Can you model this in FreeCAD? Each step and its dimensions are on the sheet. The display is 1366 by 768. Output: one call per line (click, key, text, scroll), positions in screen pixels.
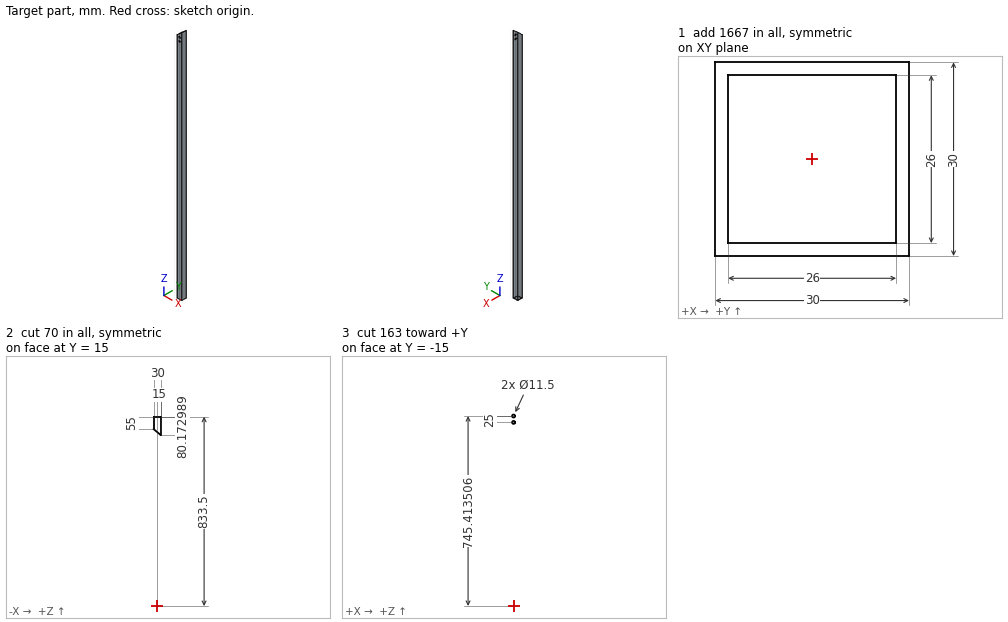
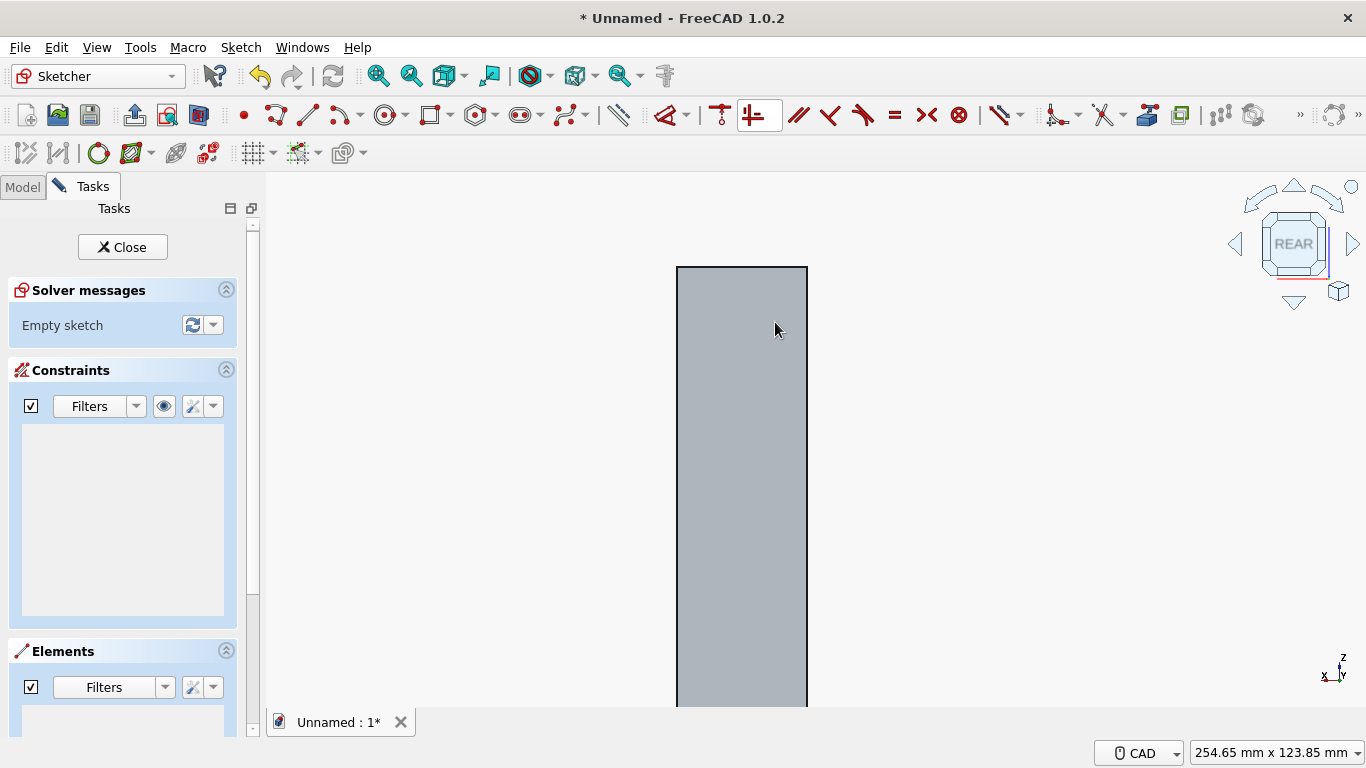
click(276, 116)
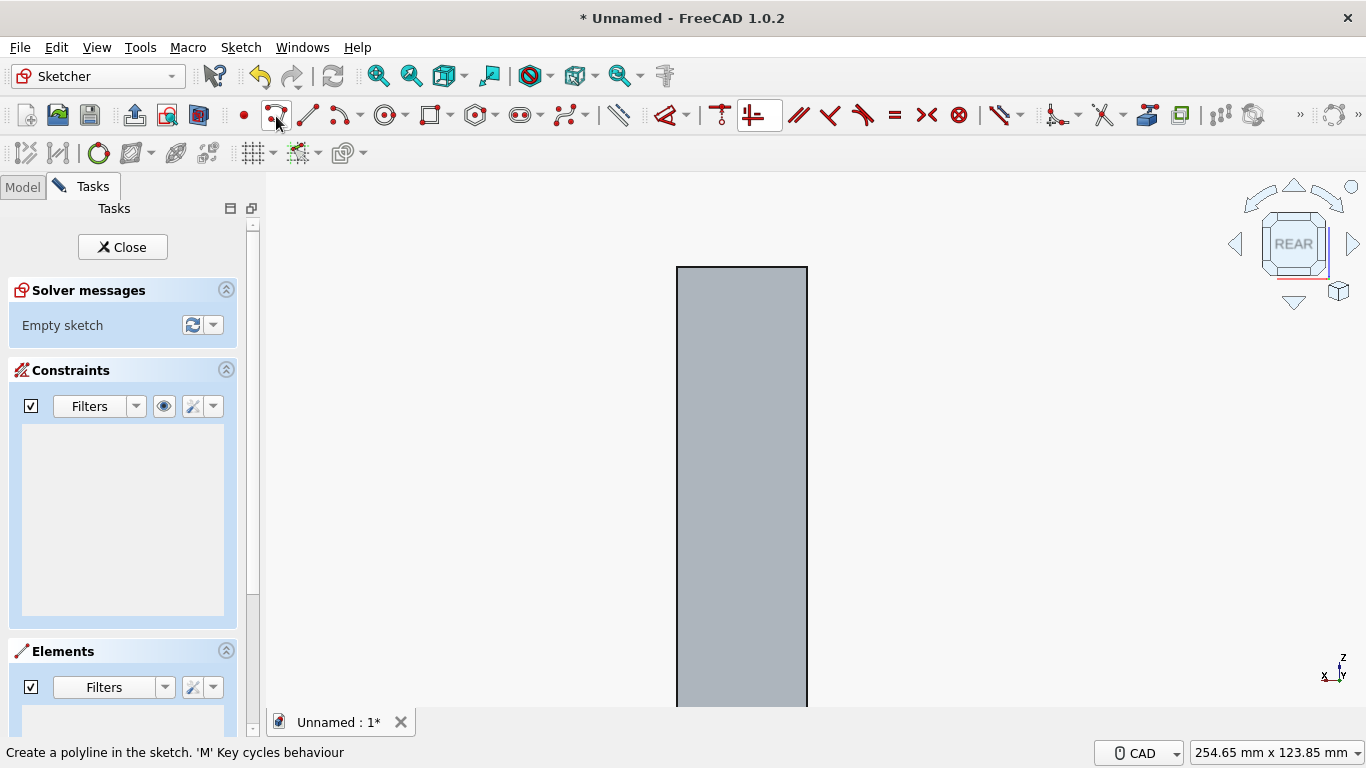
click(807, 614)
click(807, 267)
click(677, 267)
click(677, 505)
click(807, 615)
key(Escape)
key(Escape)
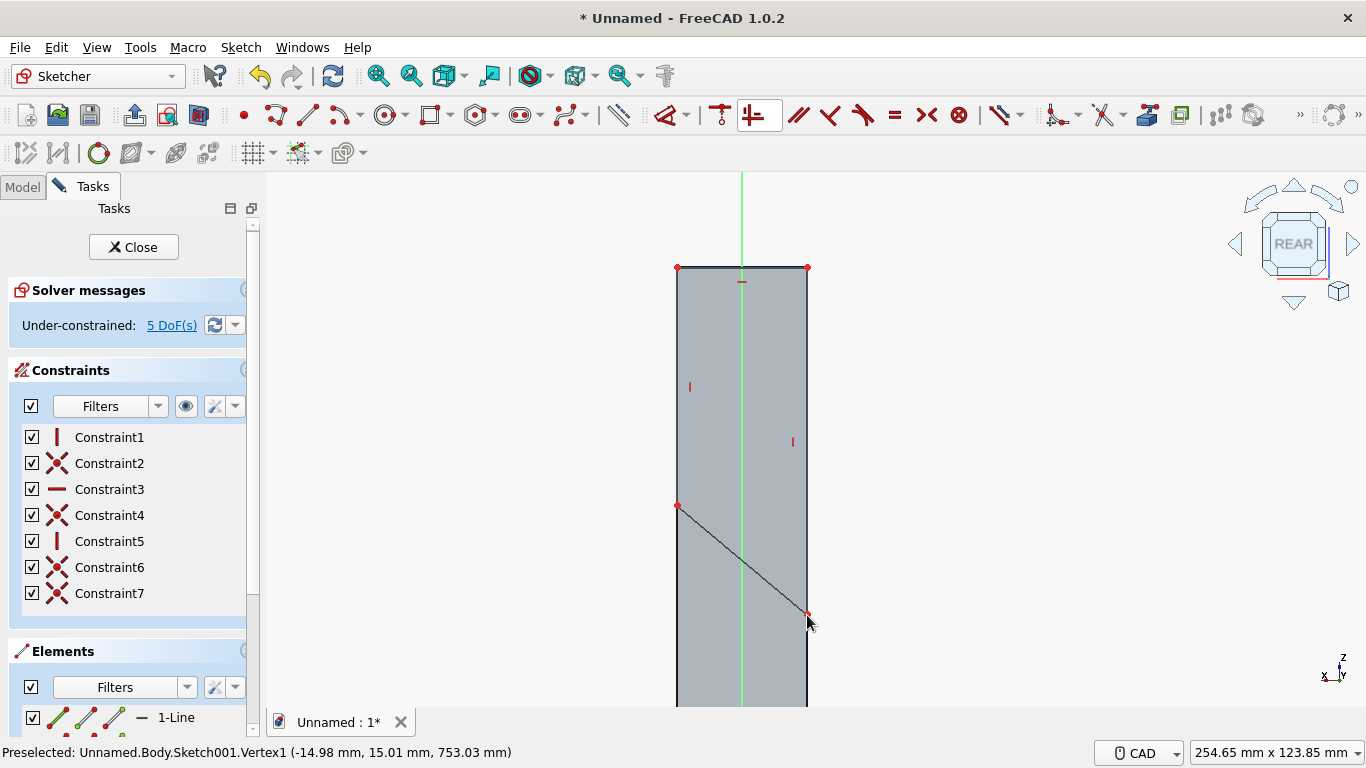
click(666, 116)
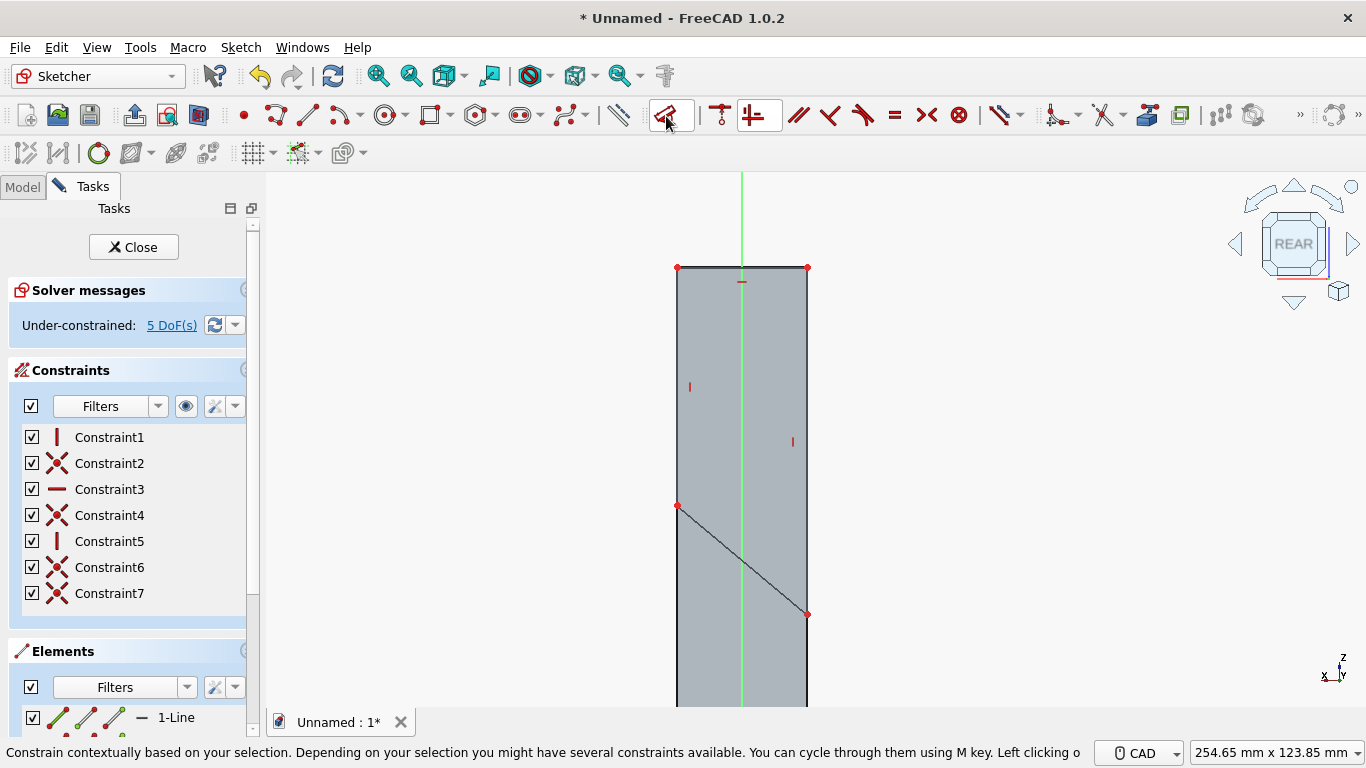
click(768, 268)
click(712, 234)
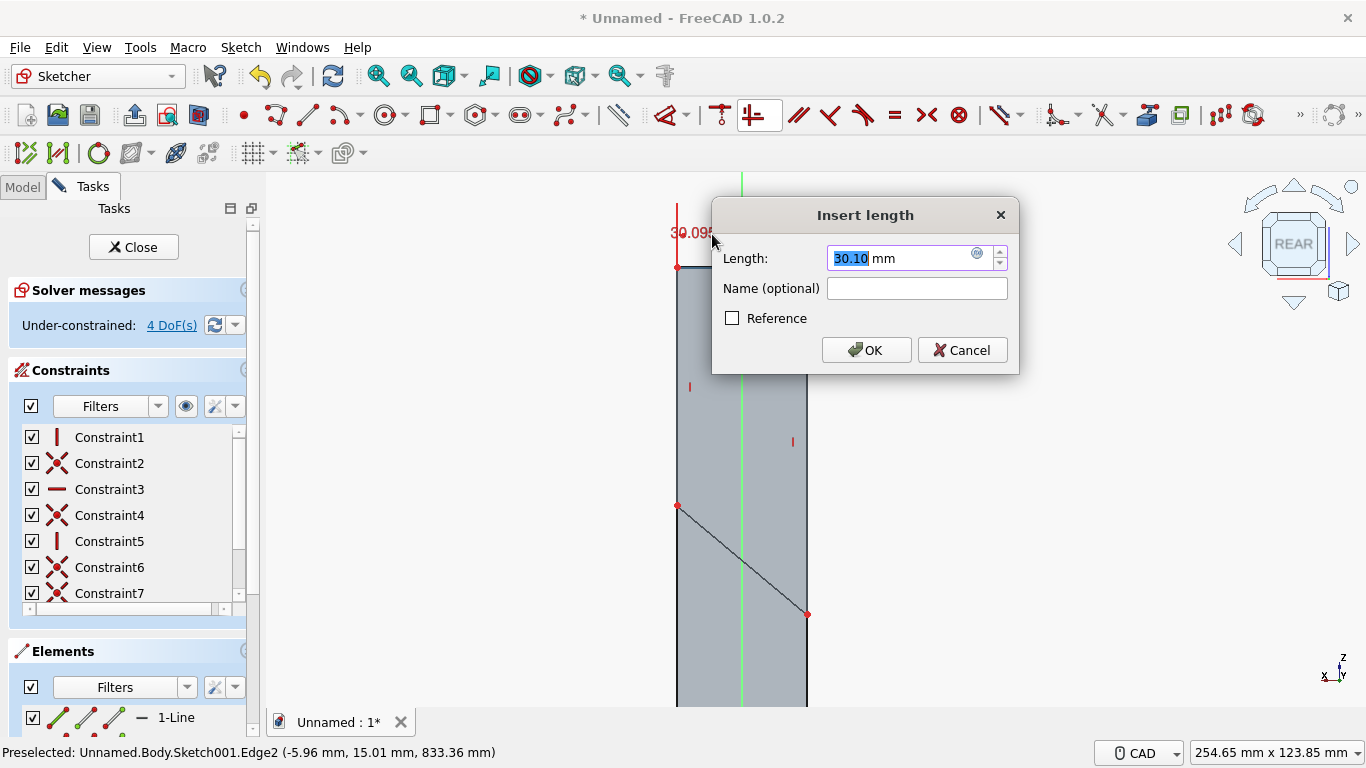
text(30)
key(Return)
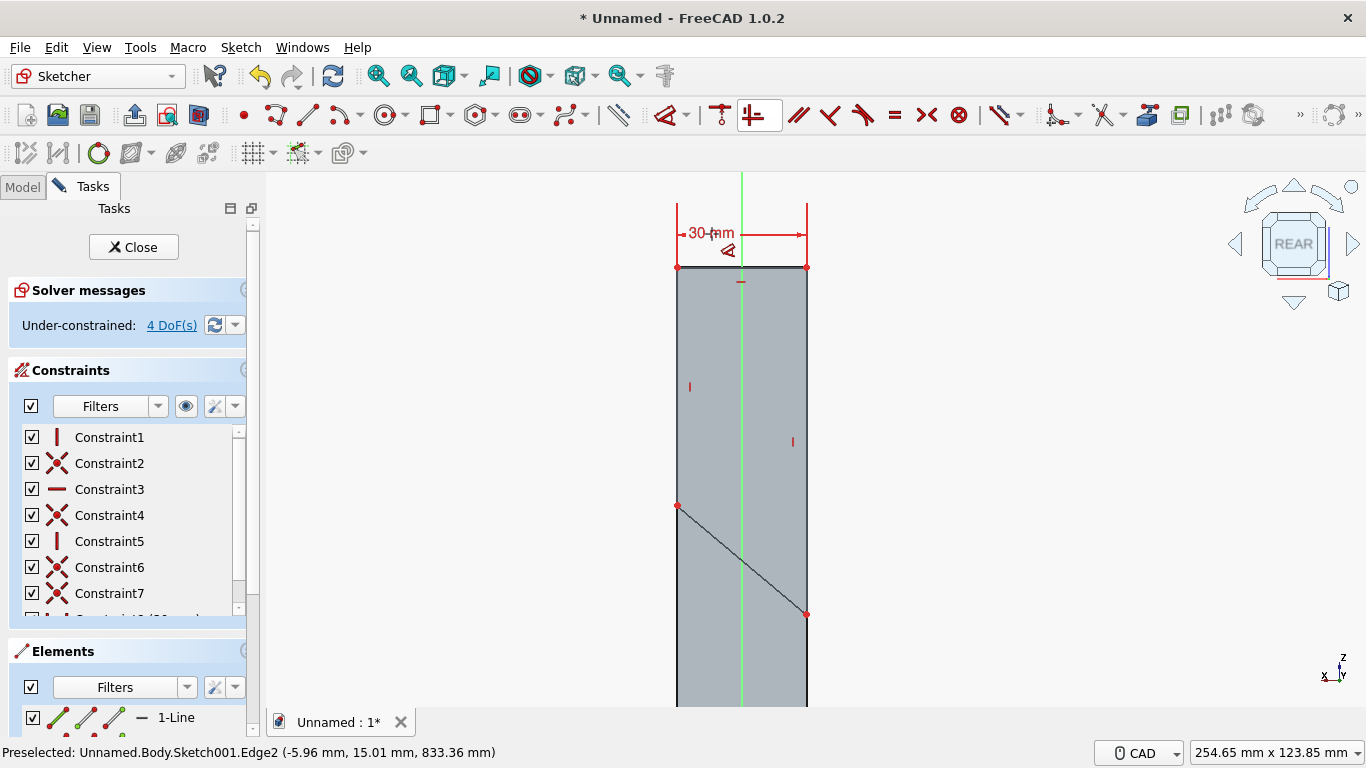
click(677, 339)
click(643, 387)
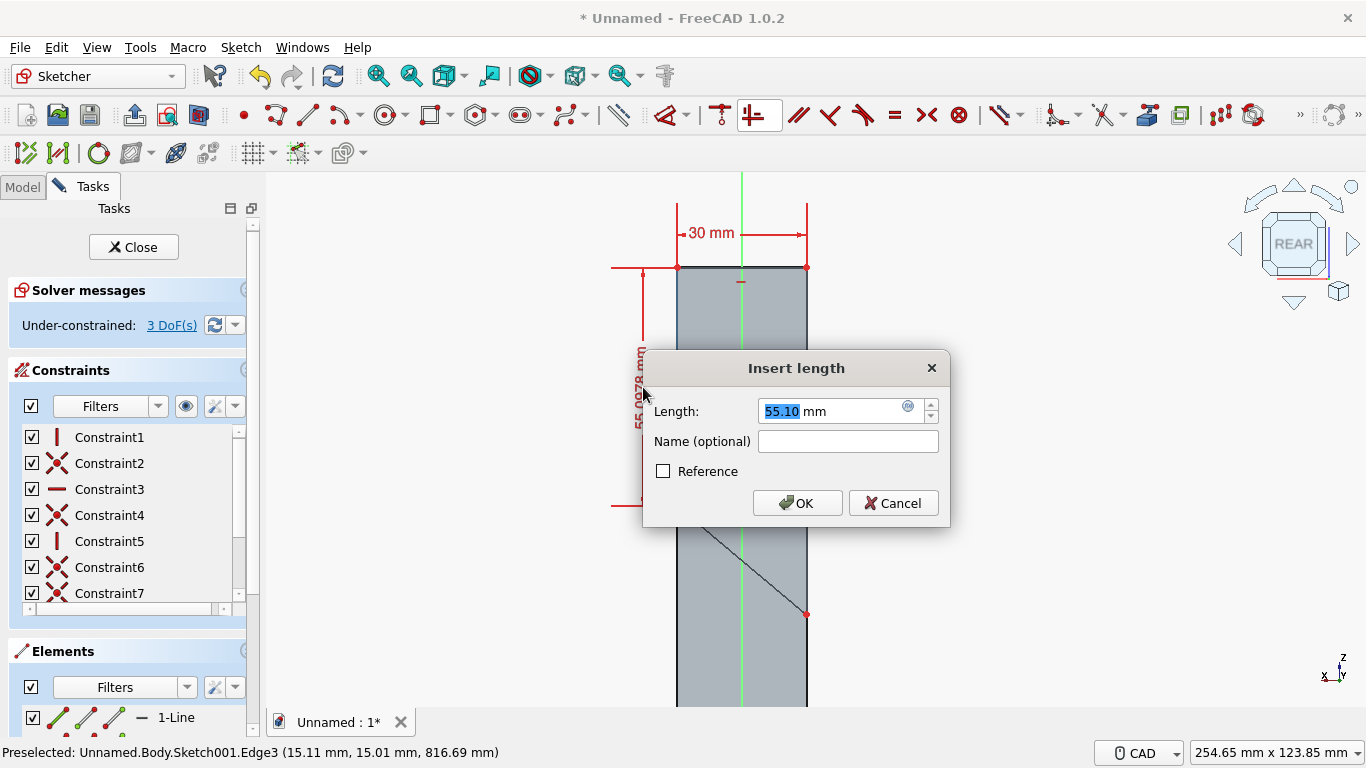
text(55)
key(Return)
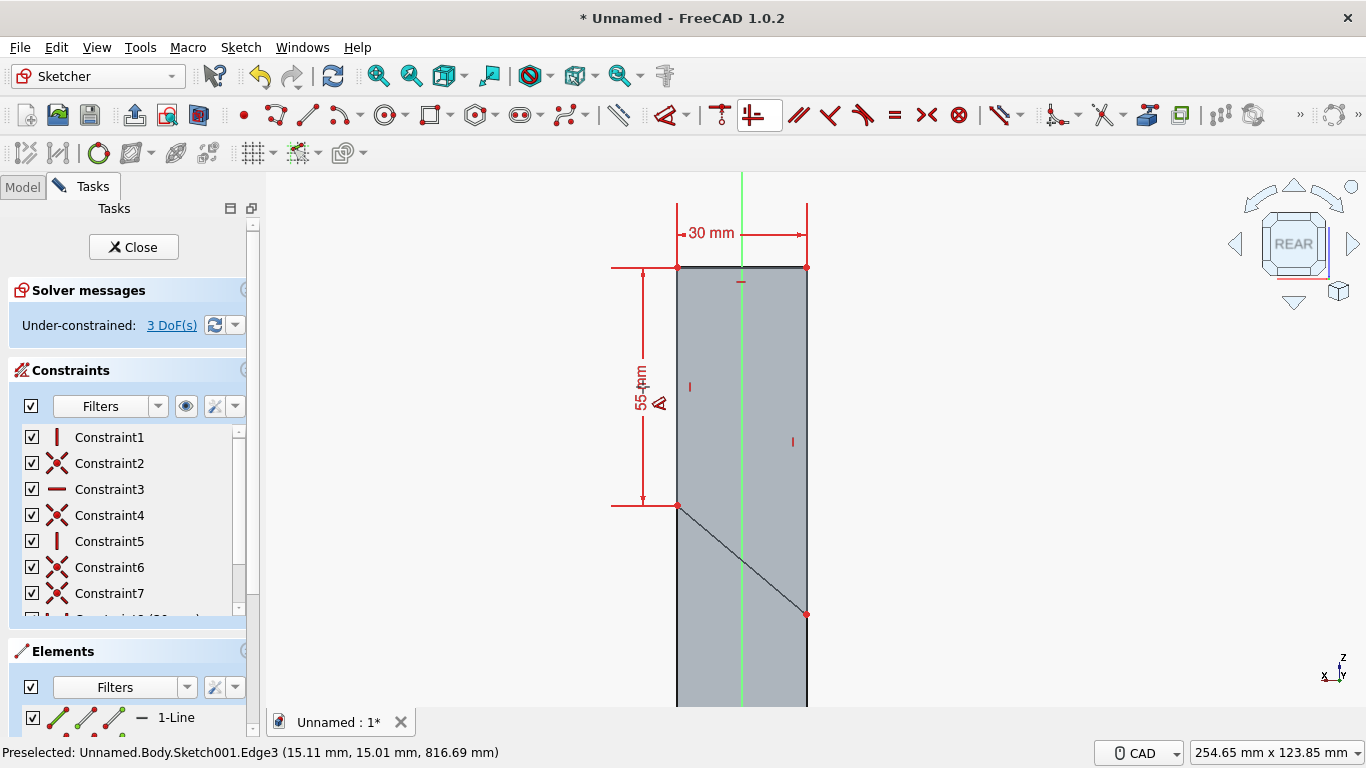
click(807, 615)
click(789, 581)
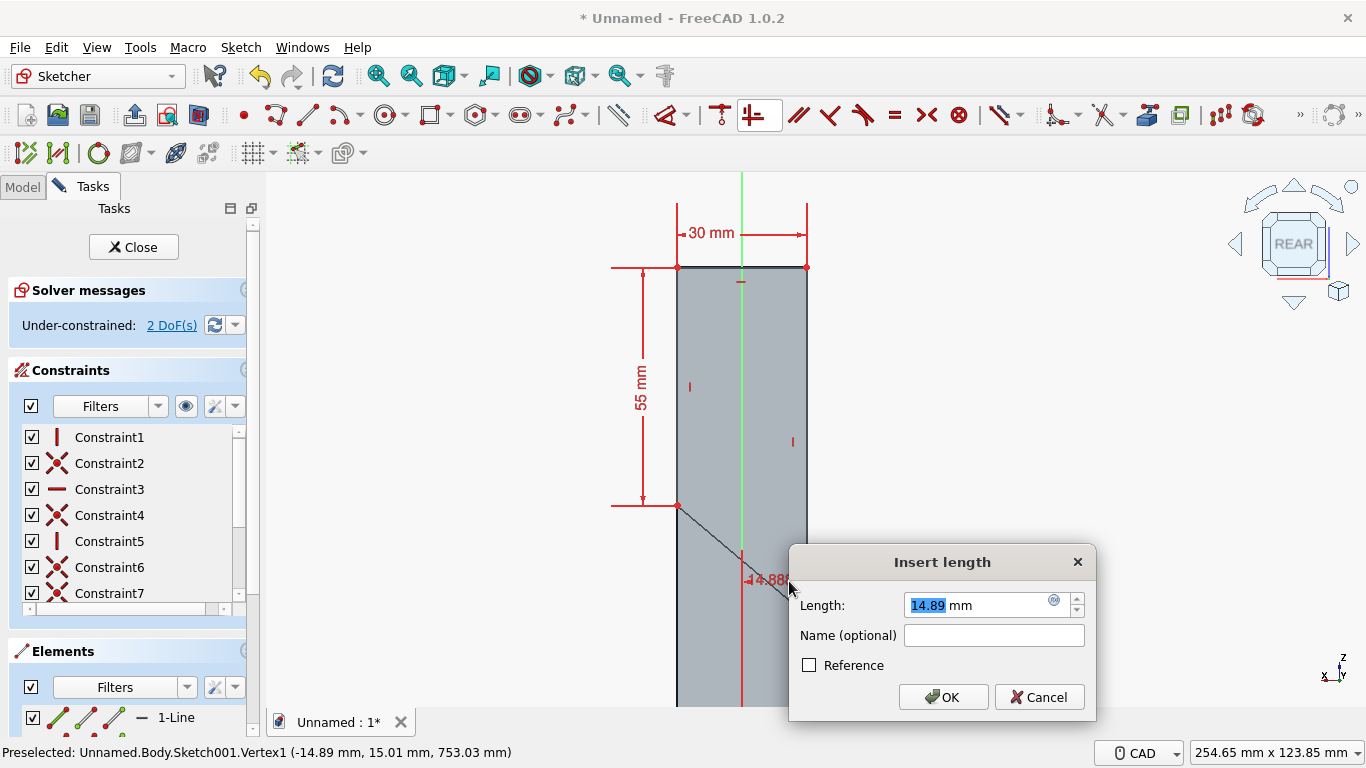
text(15)
key(Return)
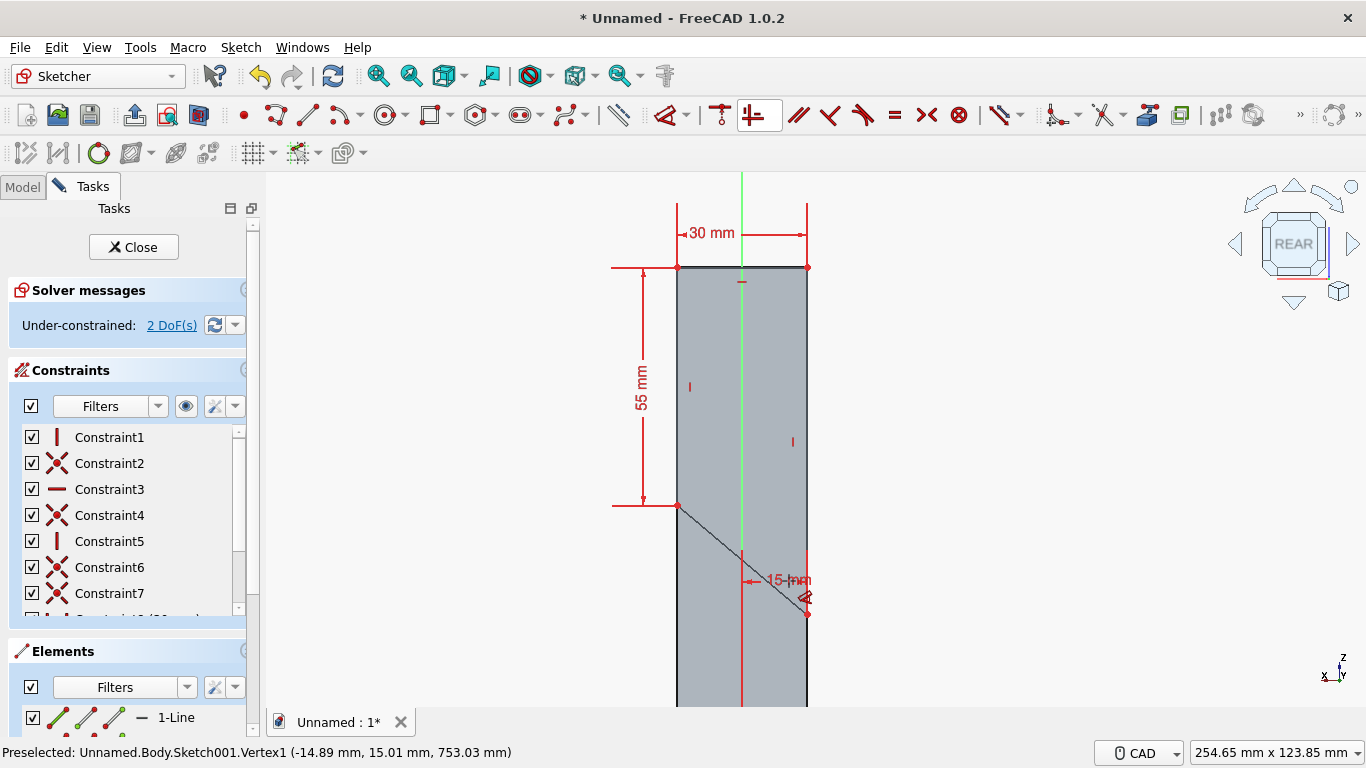
click(807, 268)
click(841, 473)